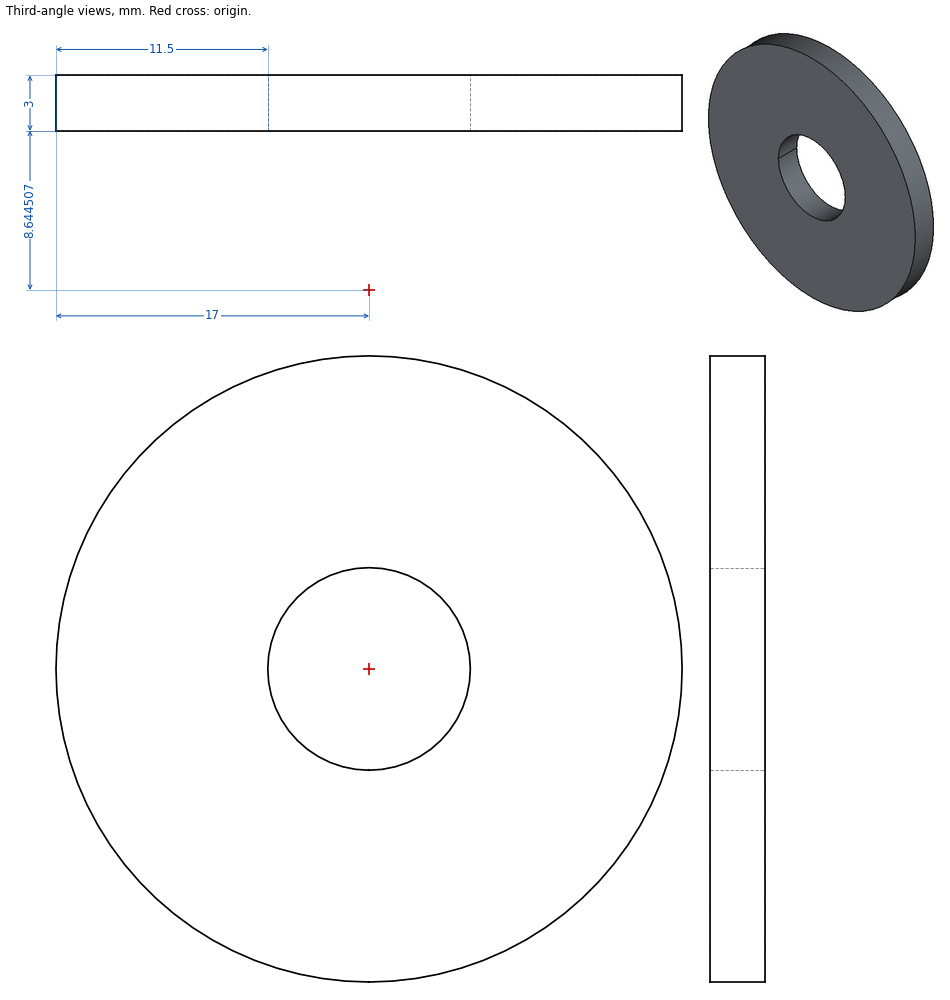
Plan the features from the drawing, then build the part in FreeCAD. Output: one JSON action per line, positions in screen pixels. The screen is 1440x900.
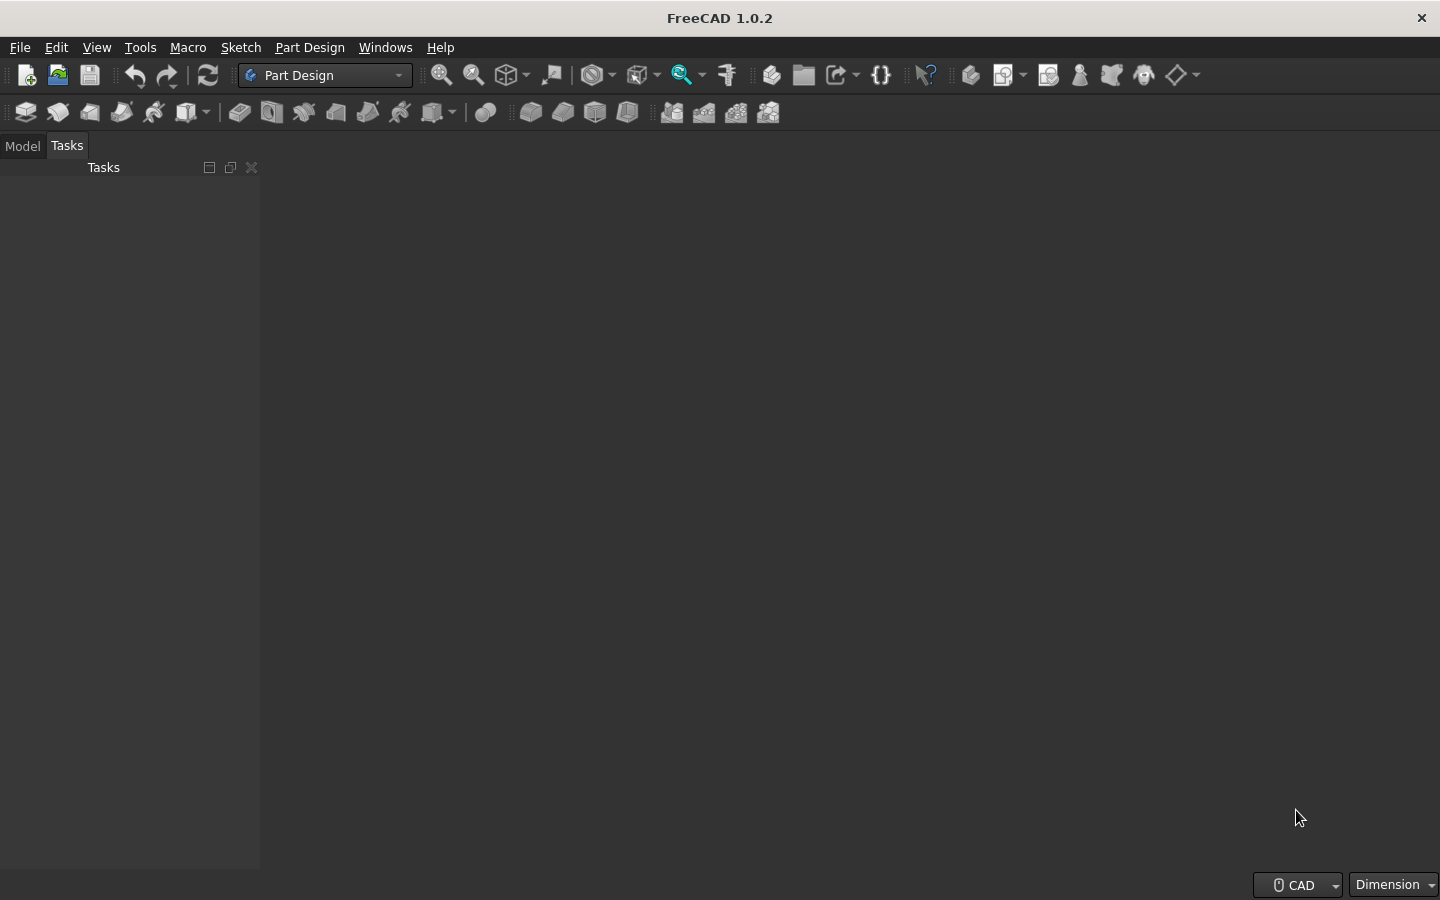
{"action": "left_click", "coordinate": [26, 76]}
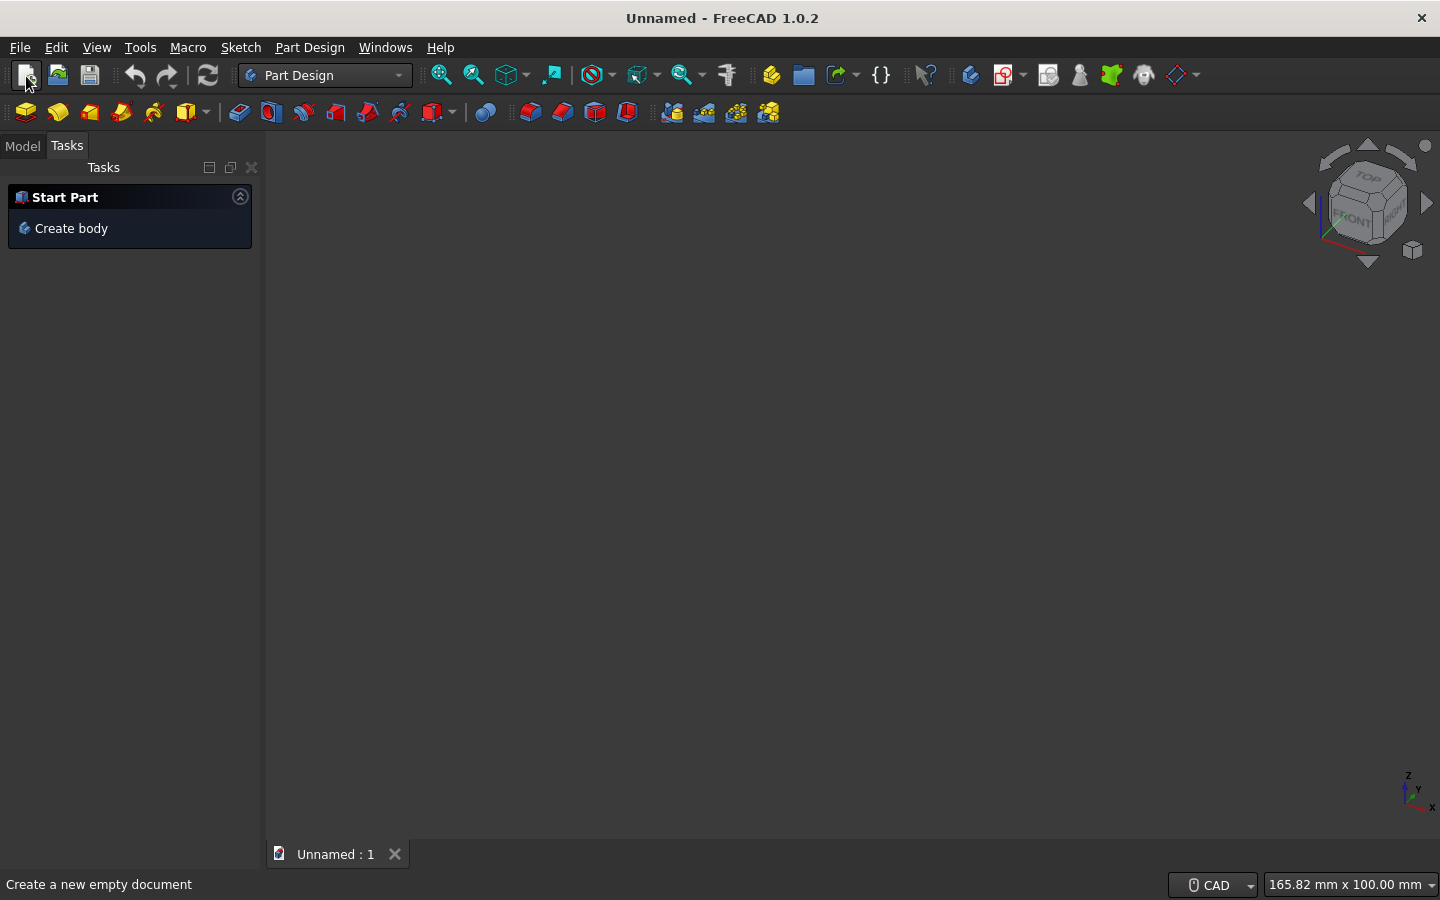
{"action": "left_click", "coordinate": [1004, 76]}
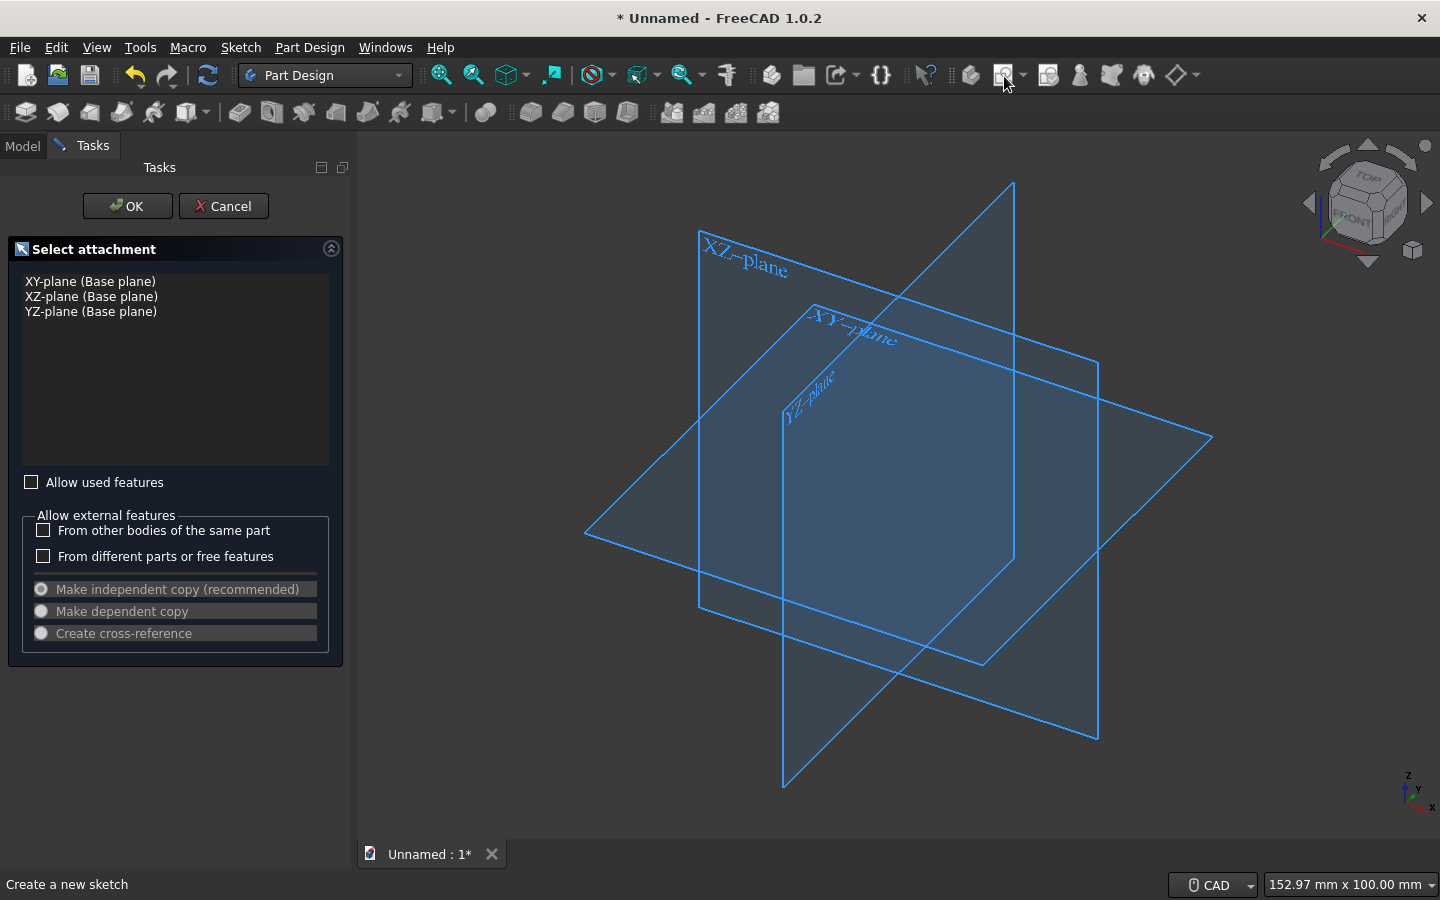
{"action": "left_click", "coordinate": [82, 282]}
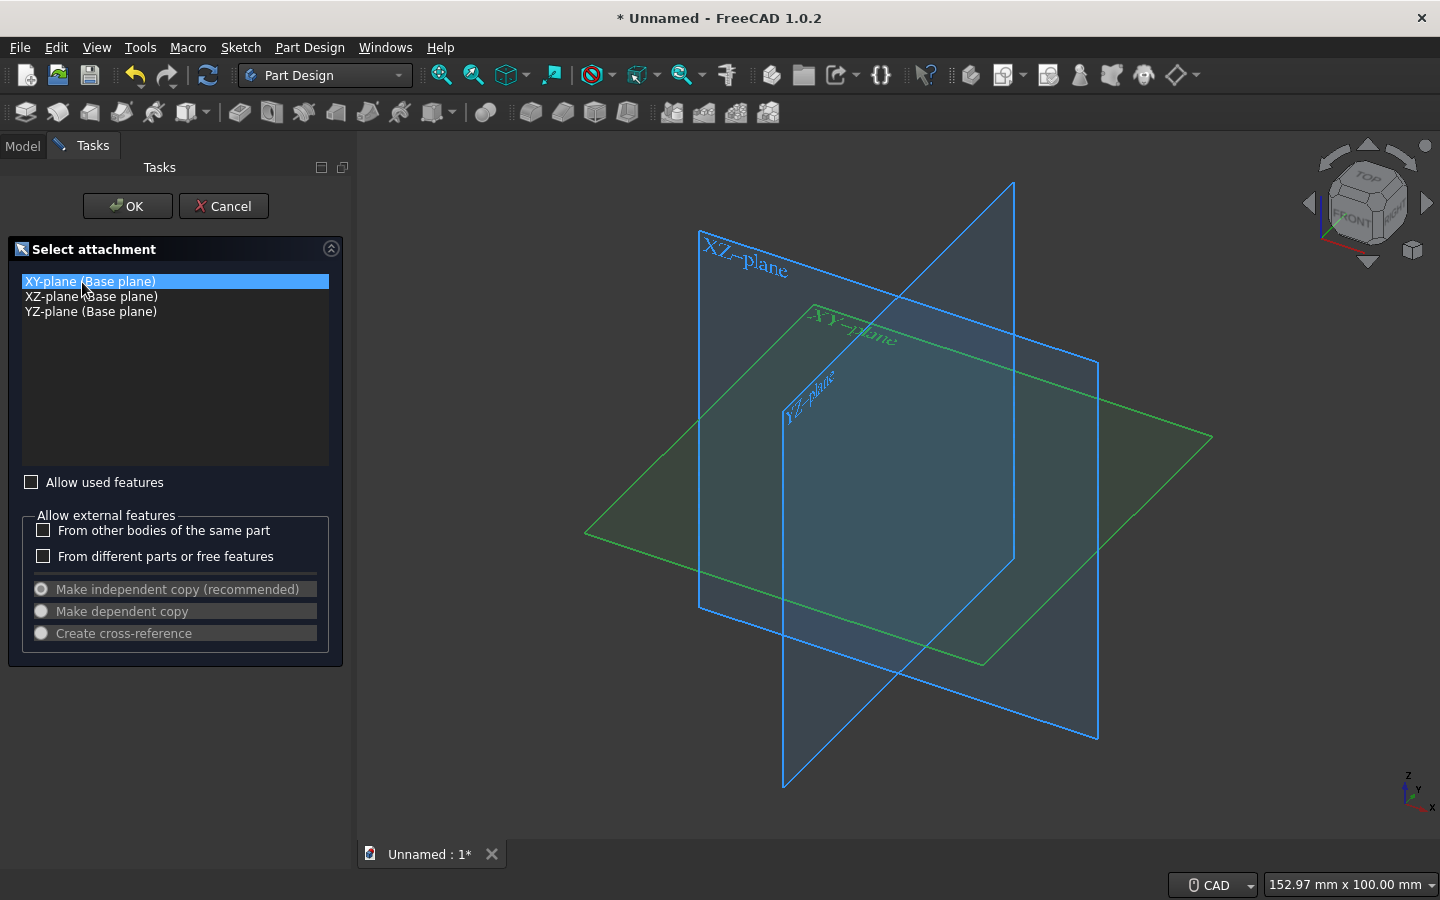
{"action": "left_click", "coordinate": [128, 206]}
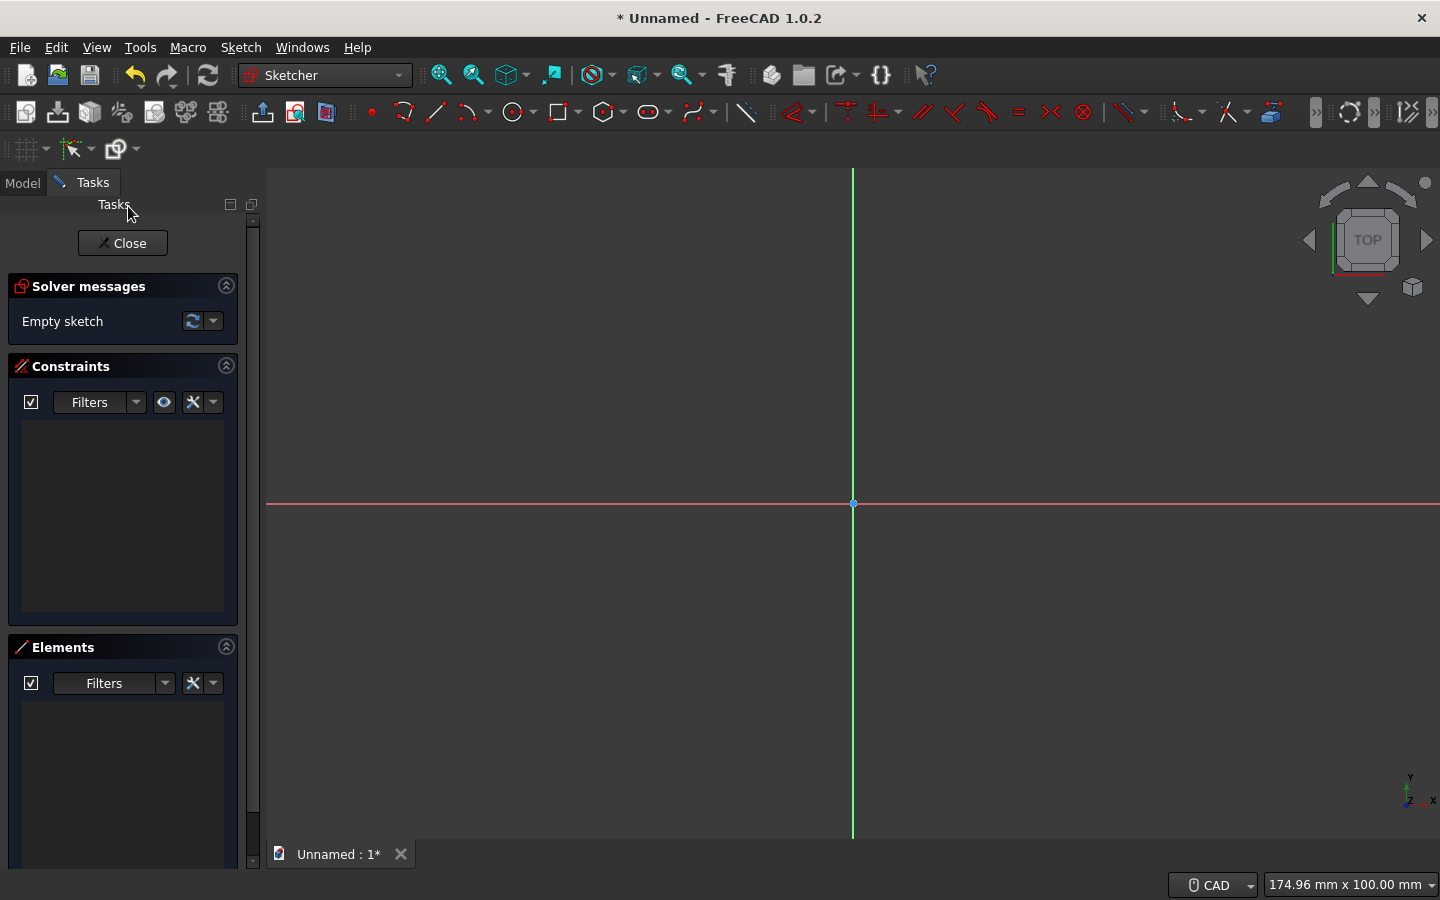
{"action": "scroll", "coordinate": [798, 457], "scroll_direction": "up", "scroll_amount": 9}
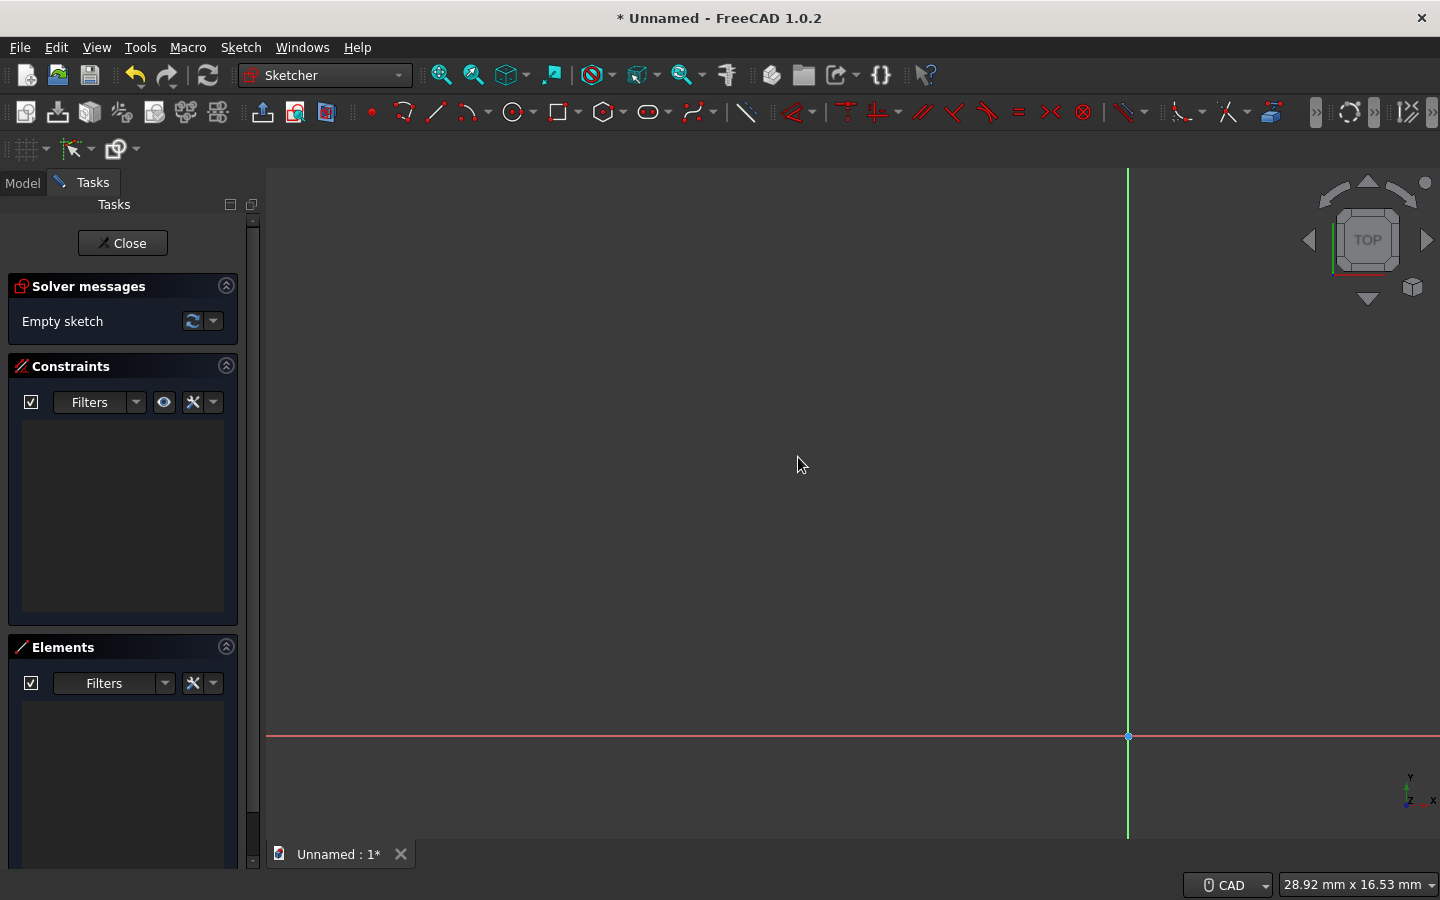
{"action": "left_click", "coordinate": [558, 112]}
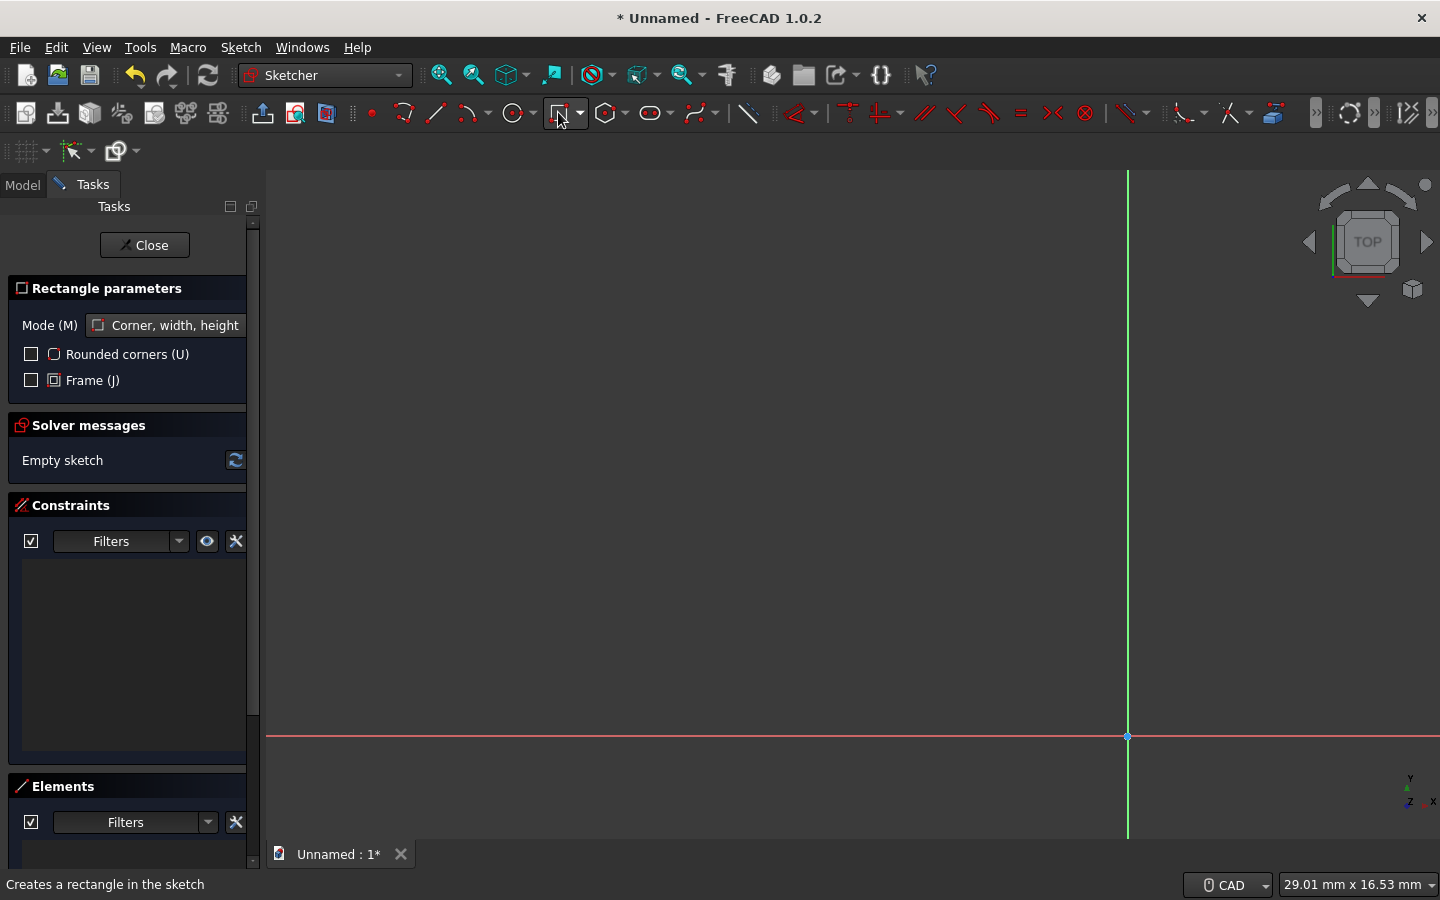
{"action": "left_click", "coordinate": [440, 265]}
{"action": "left_click", "coordinate": [905, 387]}
{"action": "key", "text": "Escape"}